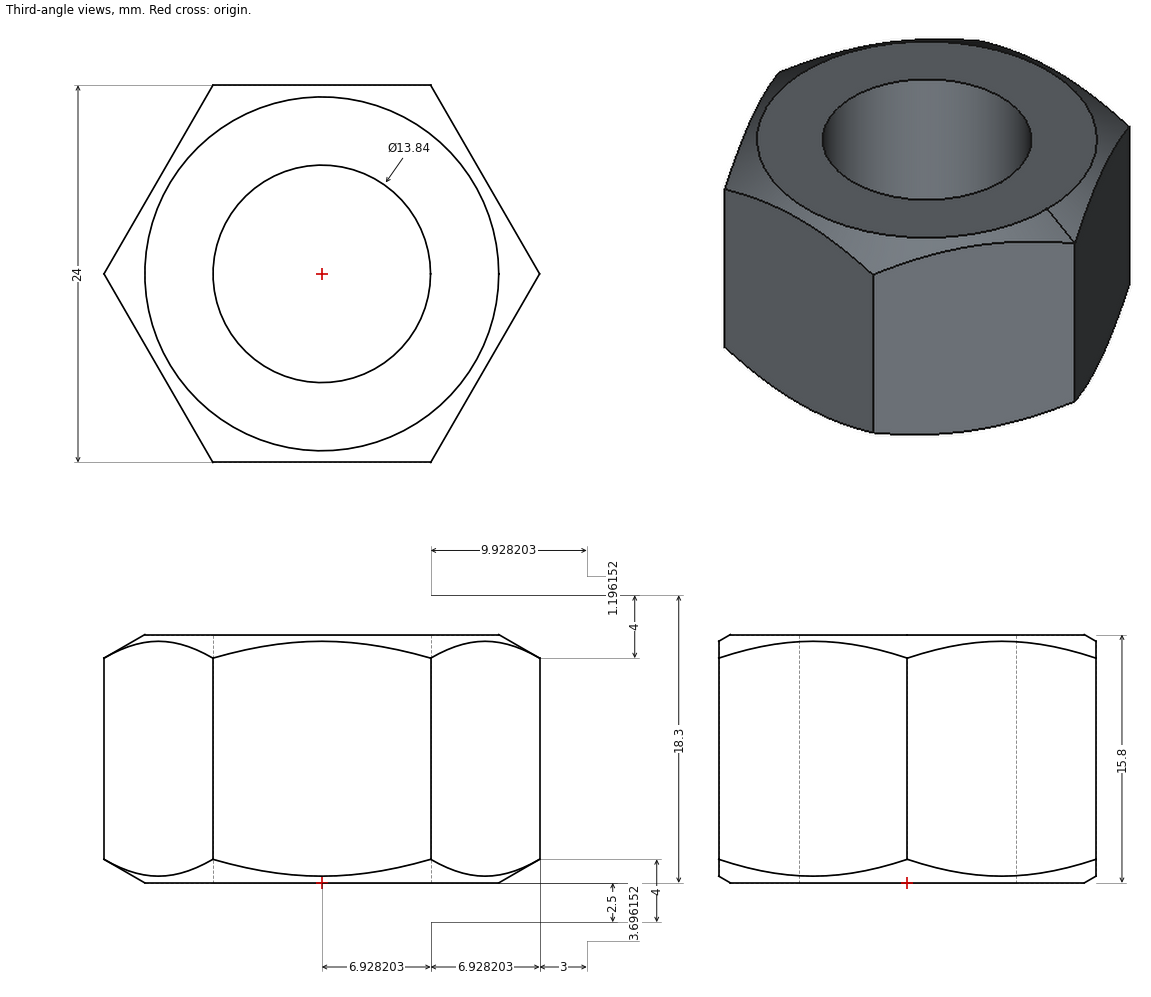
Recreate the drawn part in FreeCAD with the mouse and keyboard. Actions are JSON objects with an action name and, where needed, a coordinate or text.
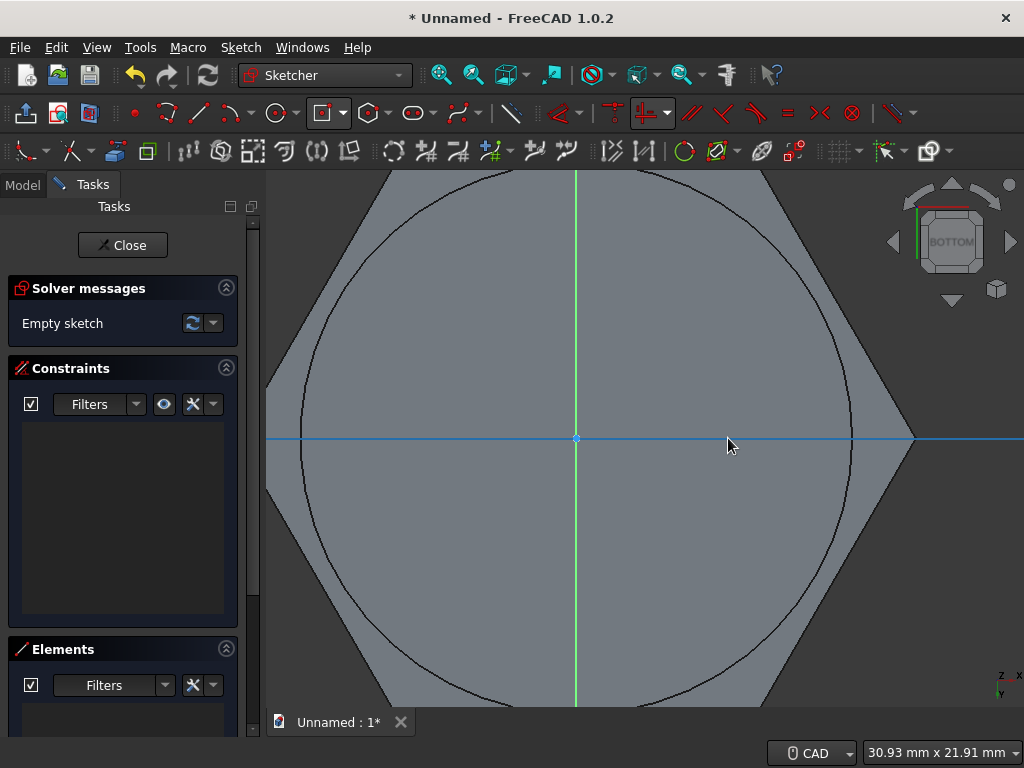
{"action": "left_click", "coordinate": [276, 114]}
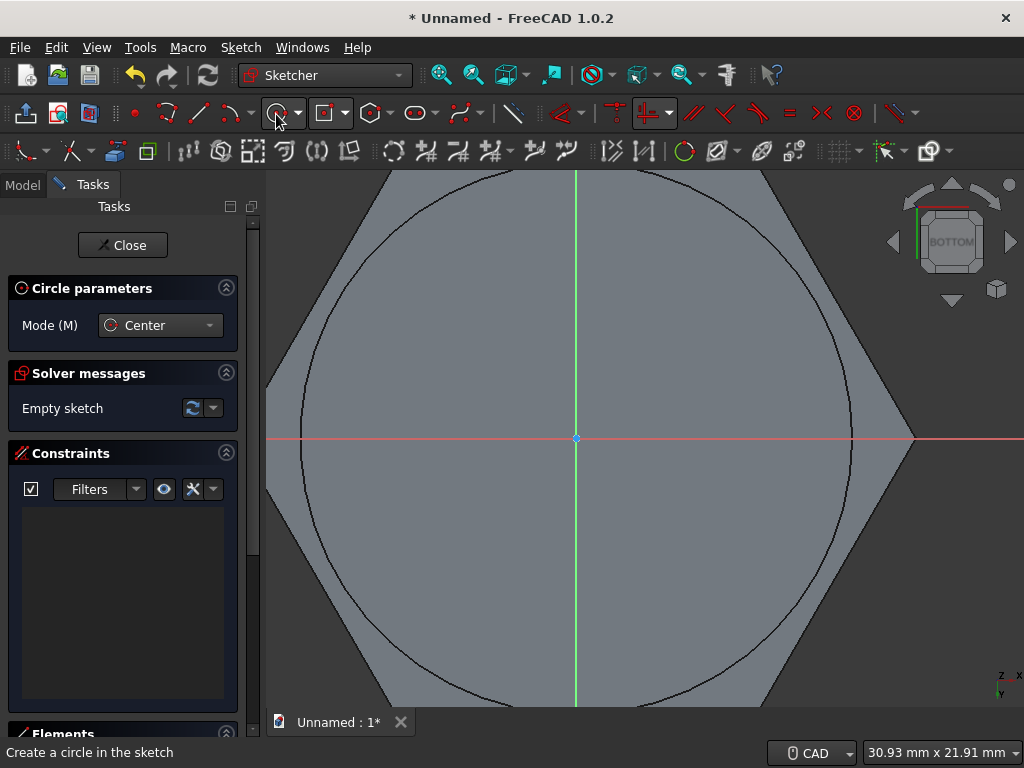
{"action": "left_click", "coordinate": [576, 438]}
{"action": "mouse_move", "coordinate": [696, 319]}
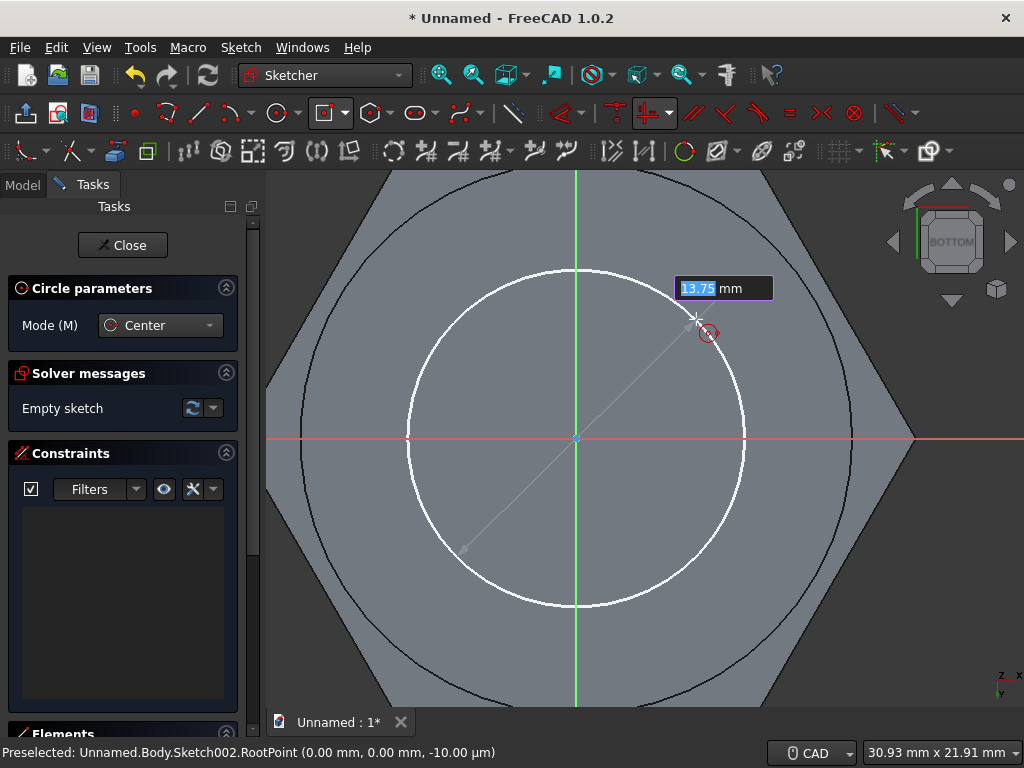
{"action": "type", "text": "13.84"}
{"action": "key", "text": "Return"}
{"action": "key", "text": "Escape"}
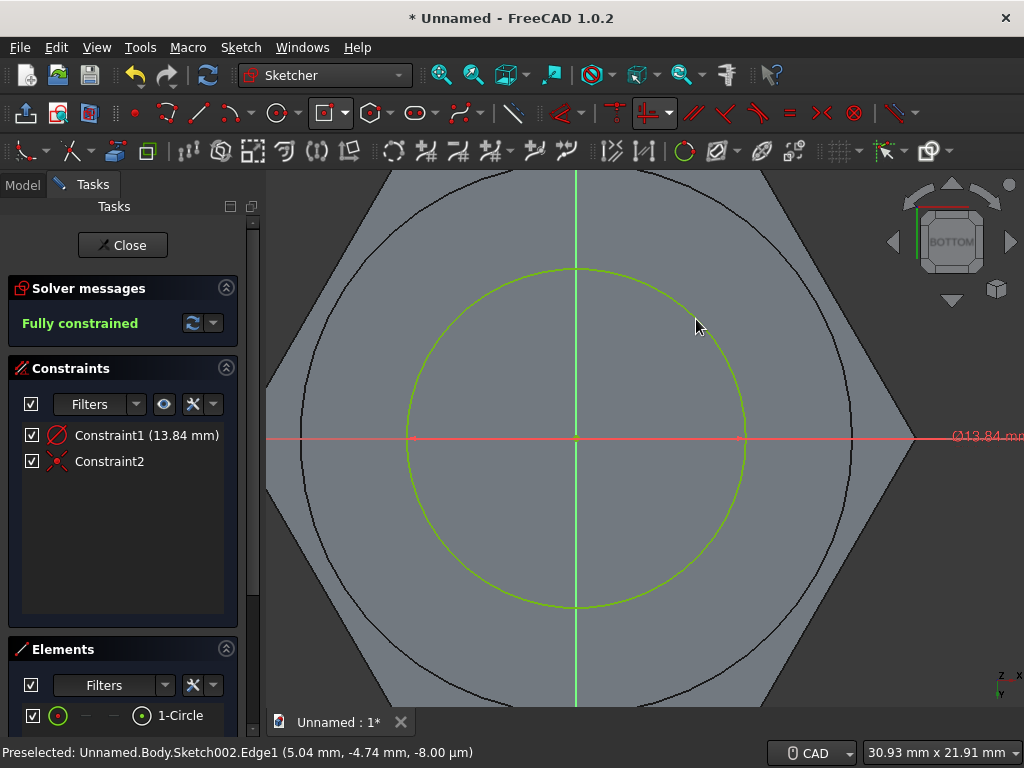
{"action": "left_click", "coordinate": [123, 245]}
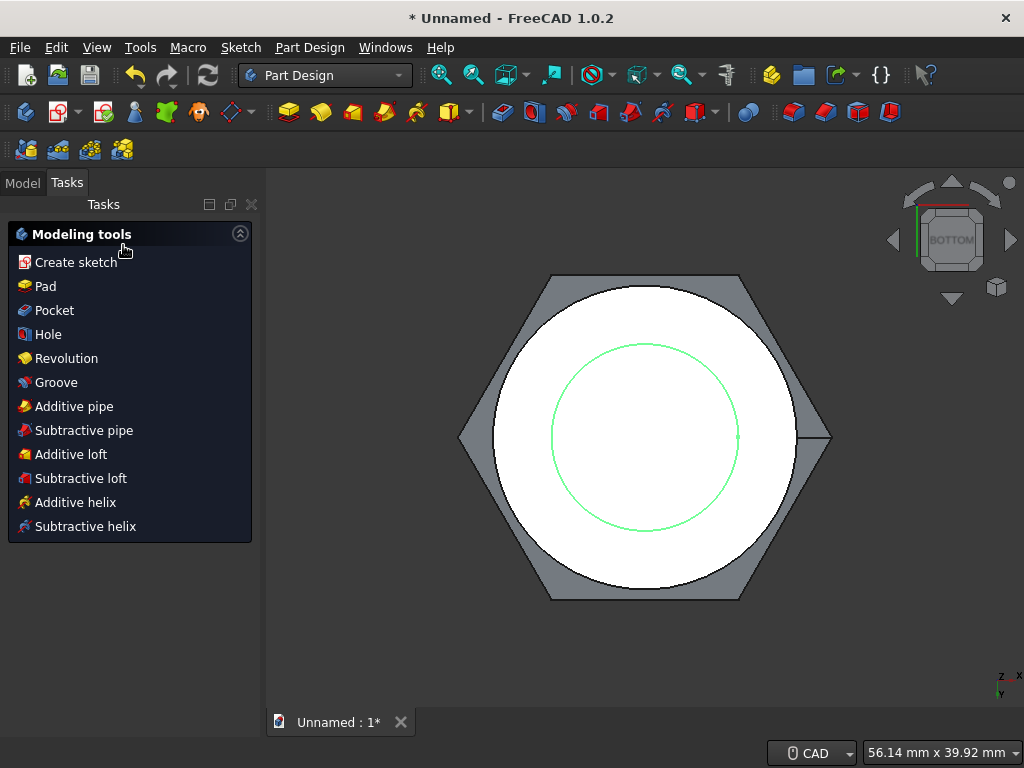
{"action": "left_click", "coordinate": [504, 112]}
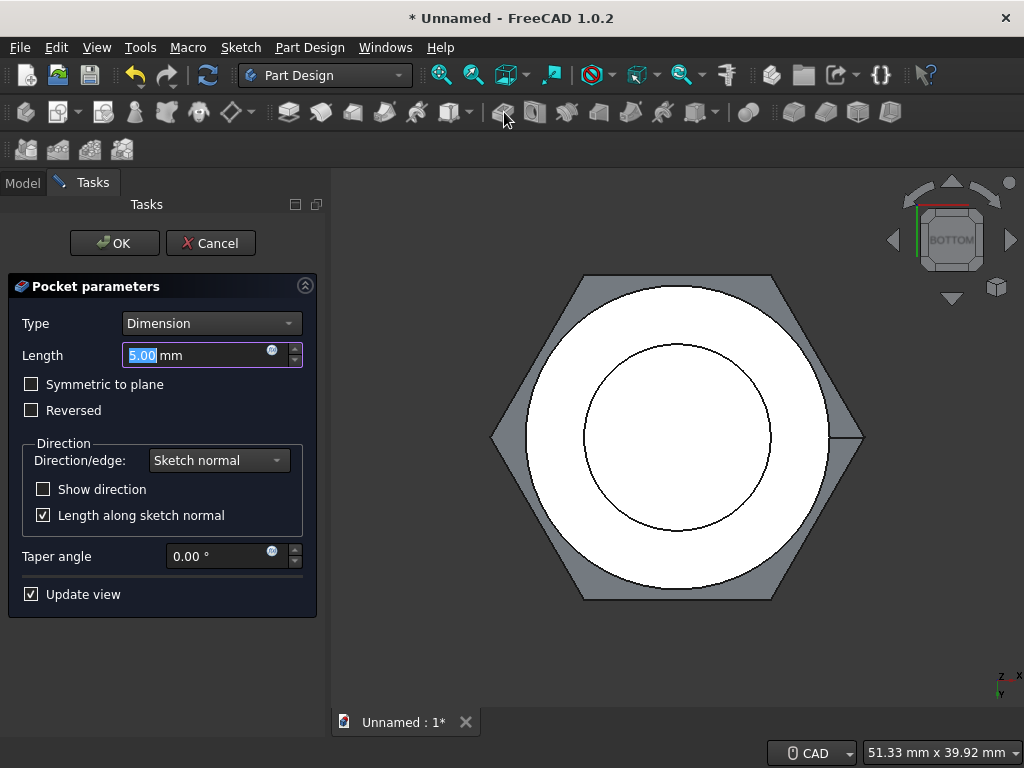
{"action": "left_click", "coordinate": [212, 324]}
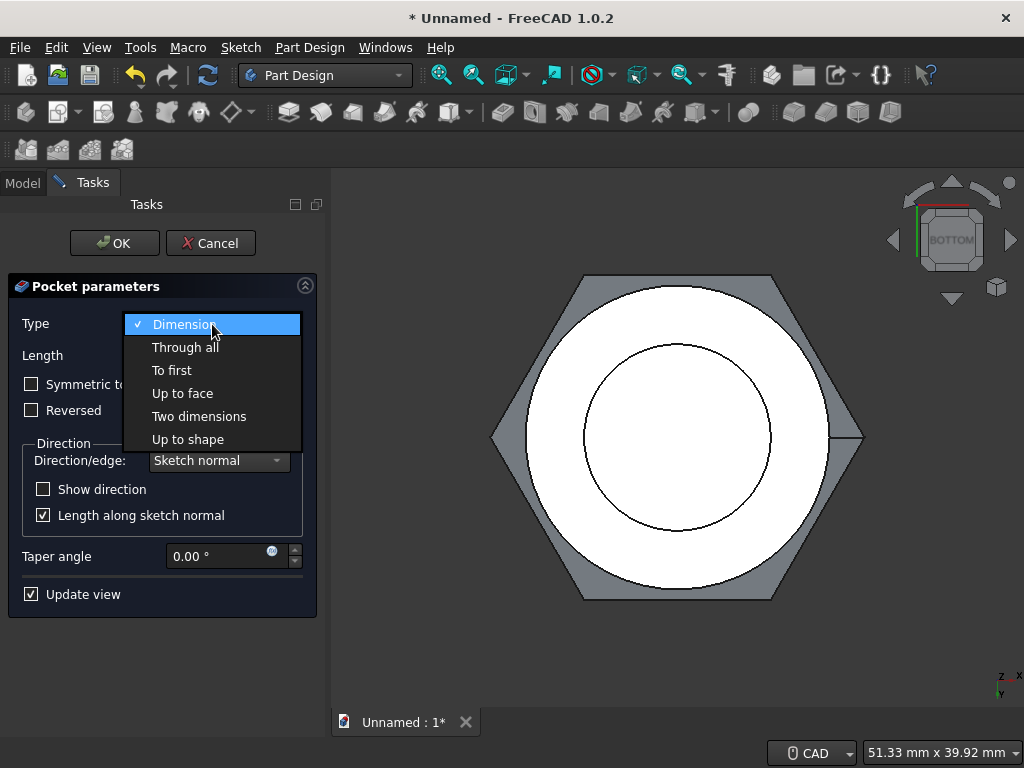
{"action": "left_click", "coordinate": [212, 348]}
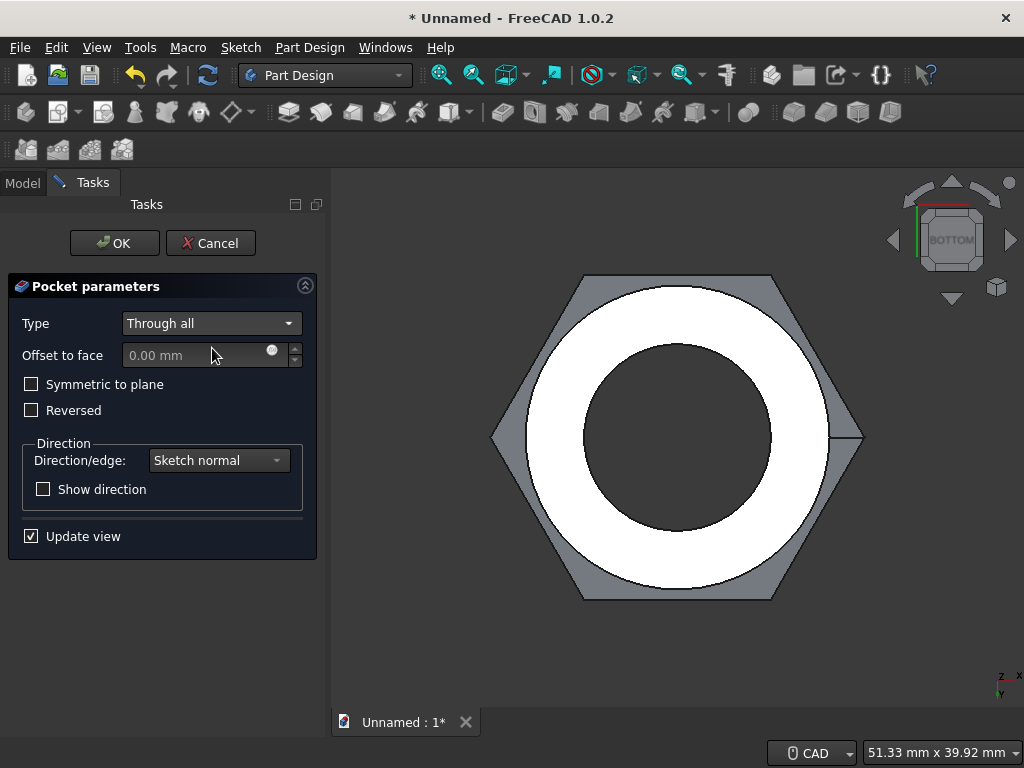
{"action": "left_click", "coordinate": [115, 243]}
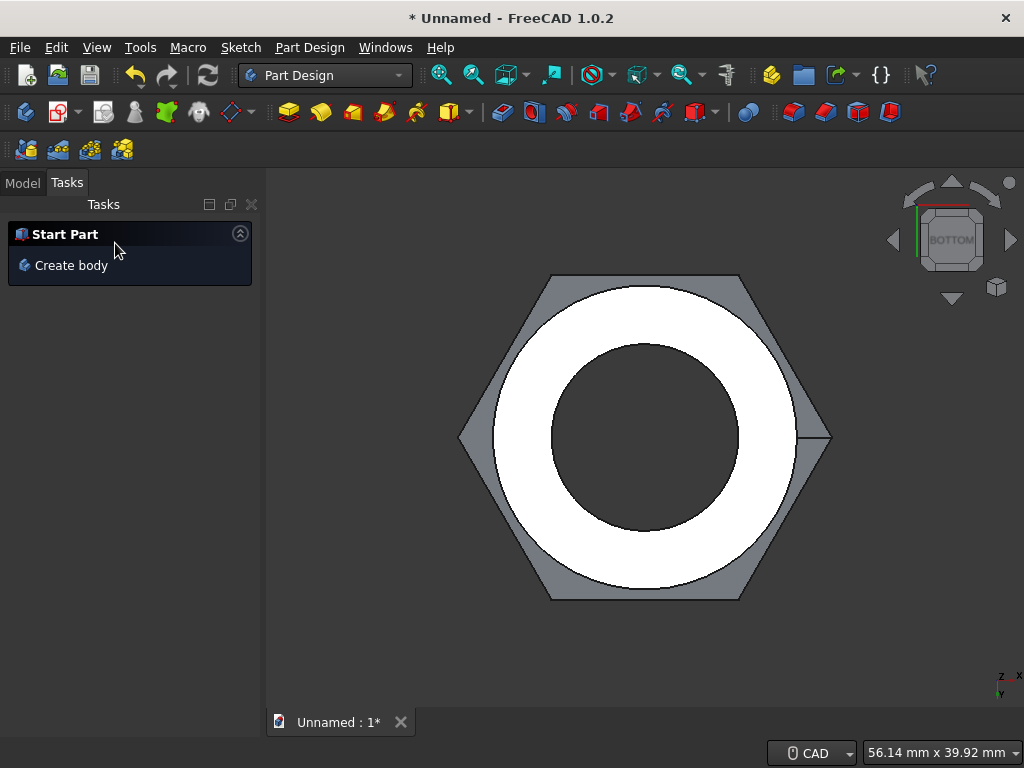
{"action": "key", "text": "0"}